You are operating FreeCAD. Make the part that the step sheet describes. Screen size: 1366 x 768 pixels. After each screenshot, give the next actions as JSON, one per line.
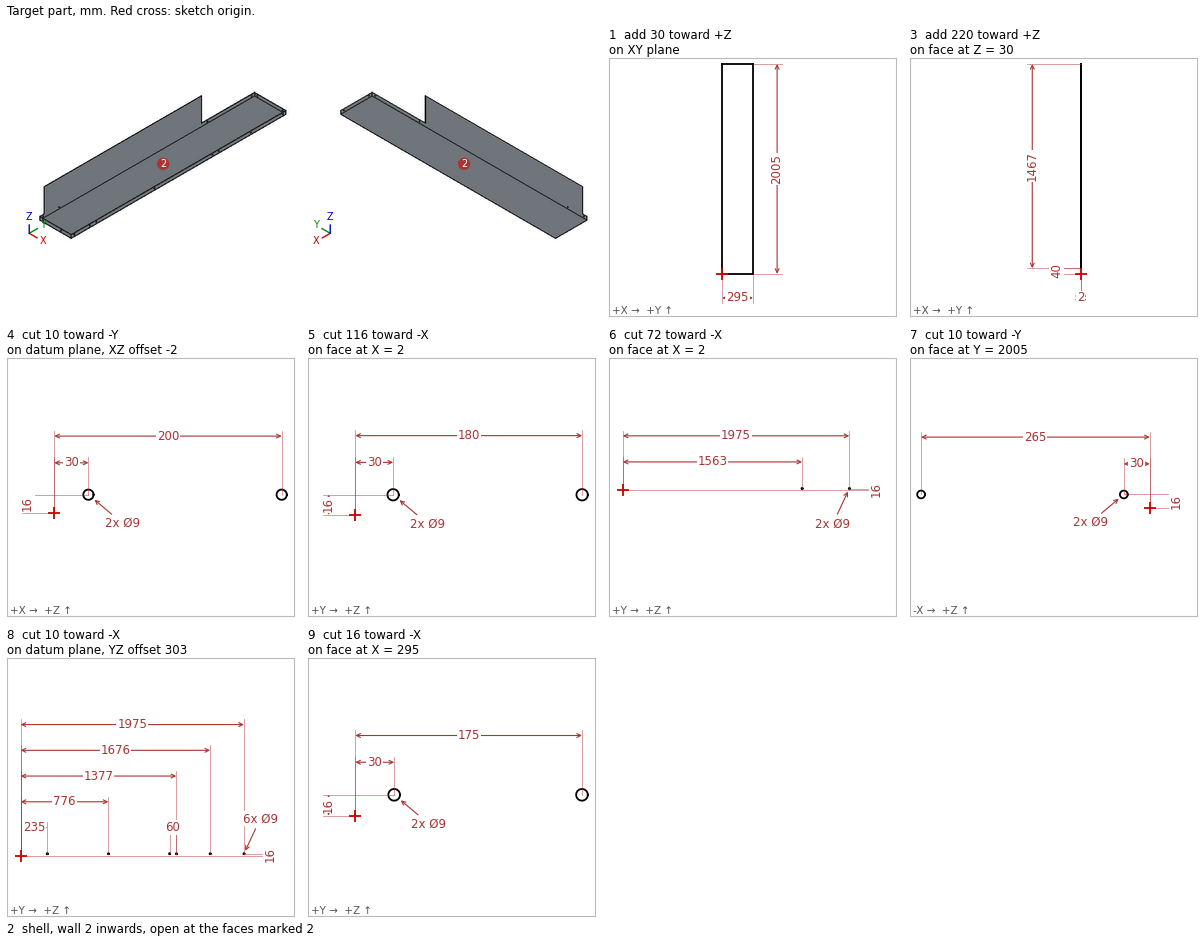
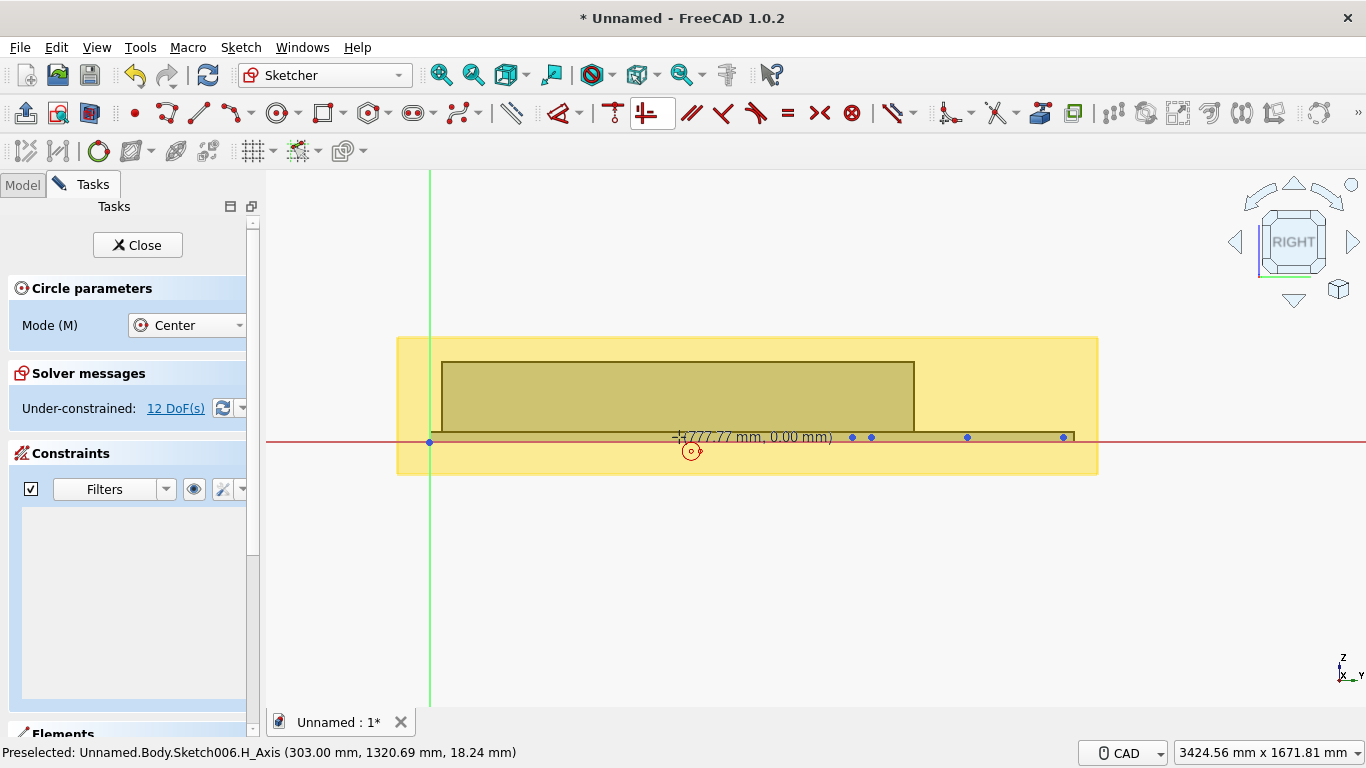
{"action": "scroll", "coordinate": [679, 437], "scroll_direction": "up", "scroll_amount": 6}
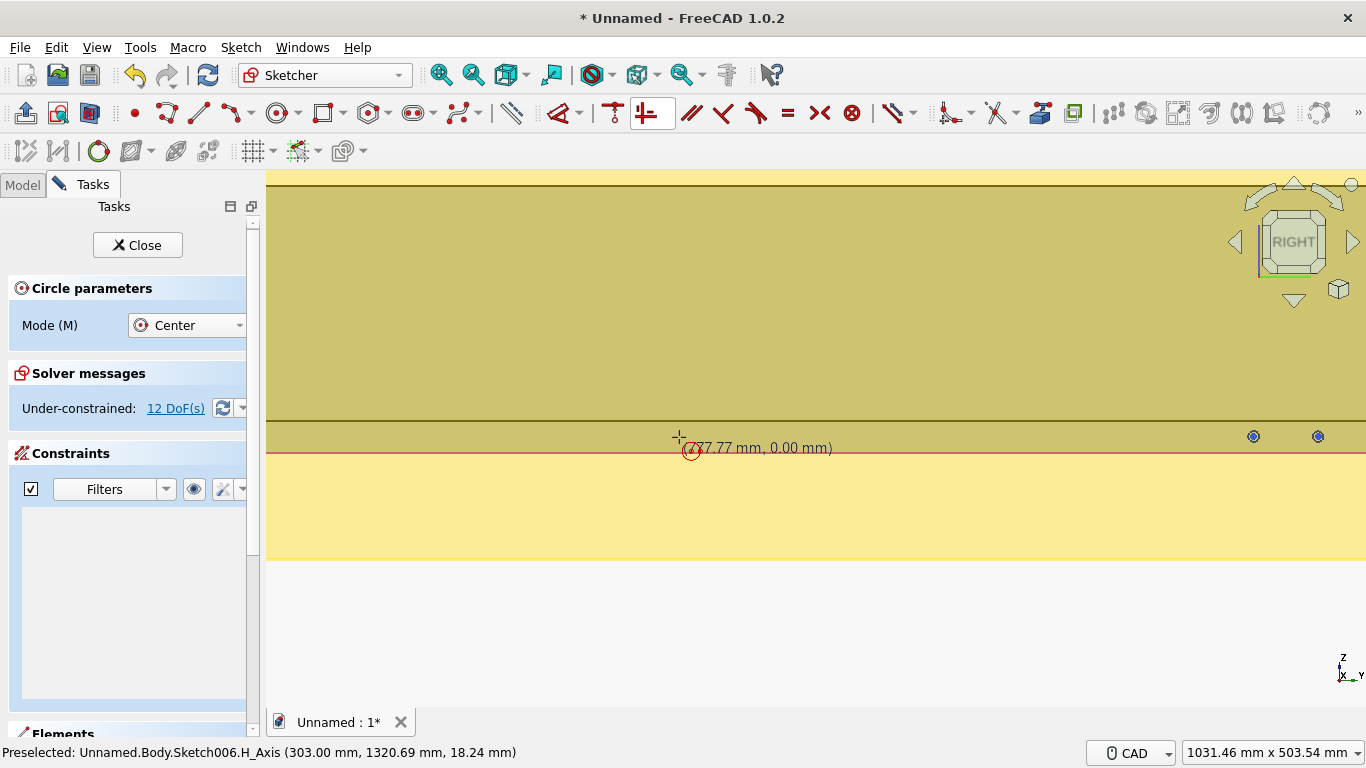
{"action": "left_click", "coordinate": [677, 436]}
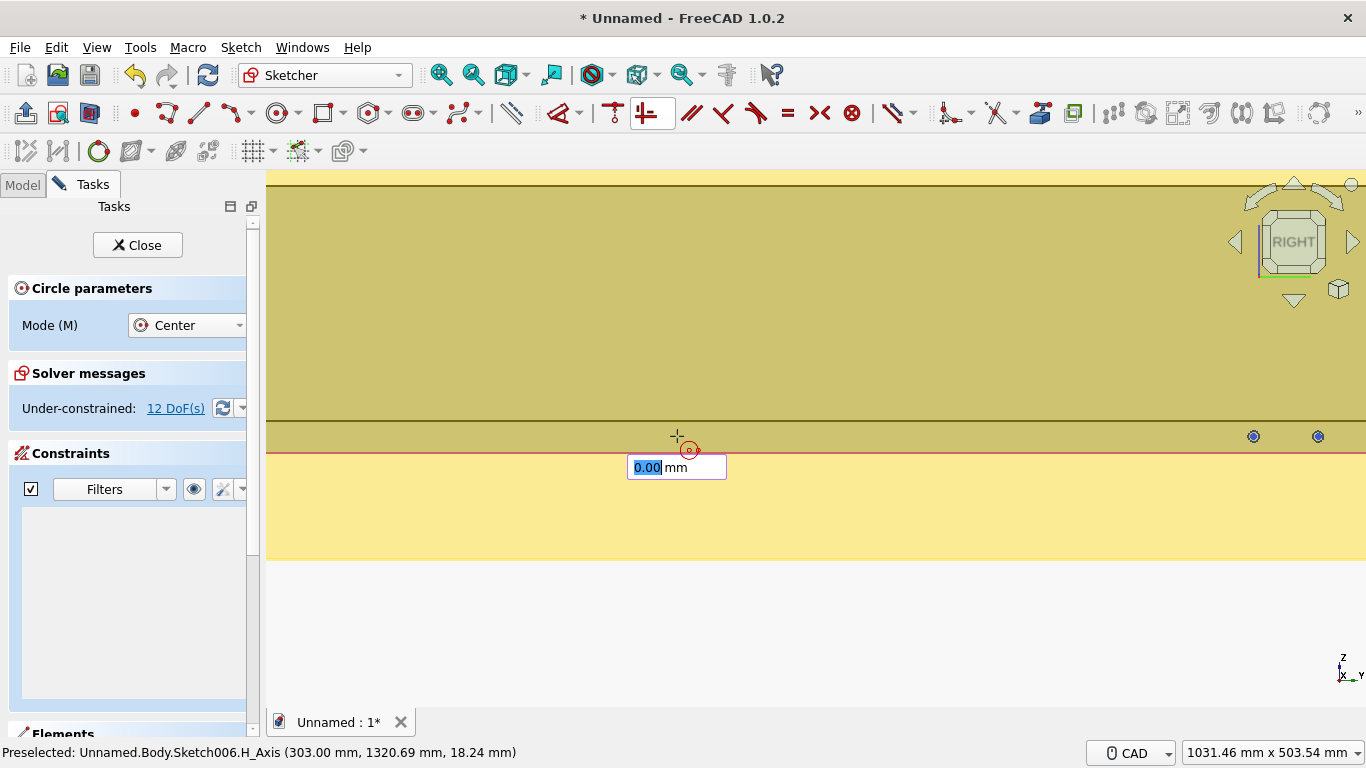
{"action": "scroll", "coordinate": [681, 432], "scroll_direction": "up", "scroll_amount": 6}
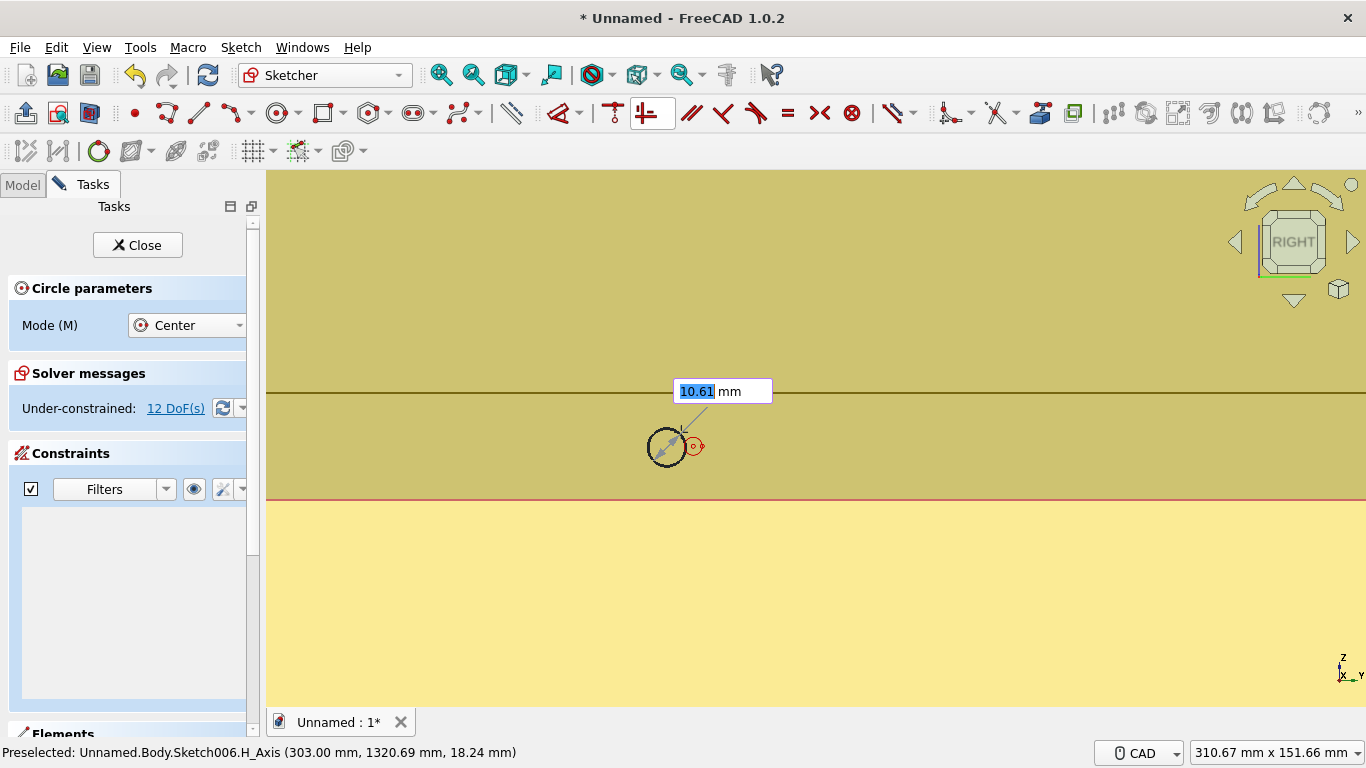
{"action": "left_click", "coordinate": [679, 432]}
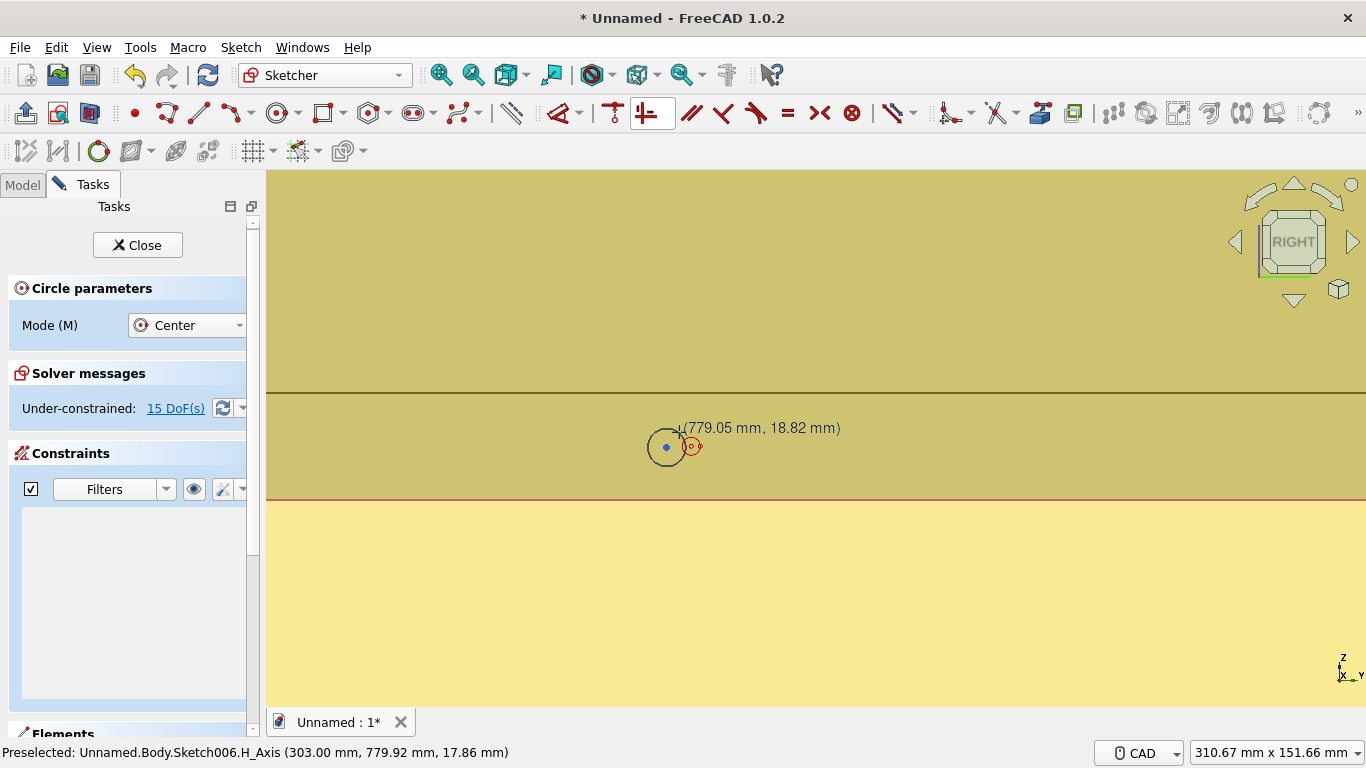
{"action": "scroll", "coordinate": [680, 436], "scroll_direction": "down", "scroll_amount": 12}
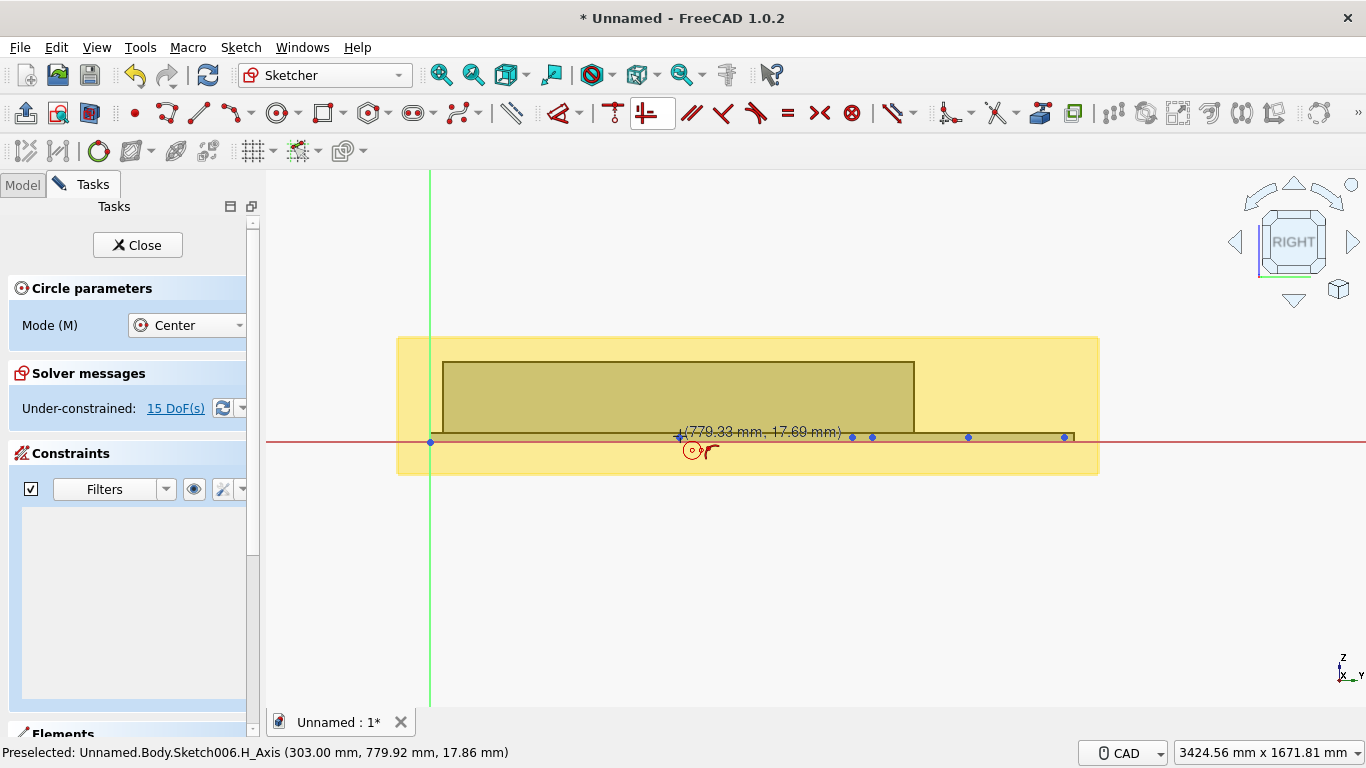
{"action": "scroll", "coordinate": [505, 437], "scroll_direction": "up", "scroll_amount": 14}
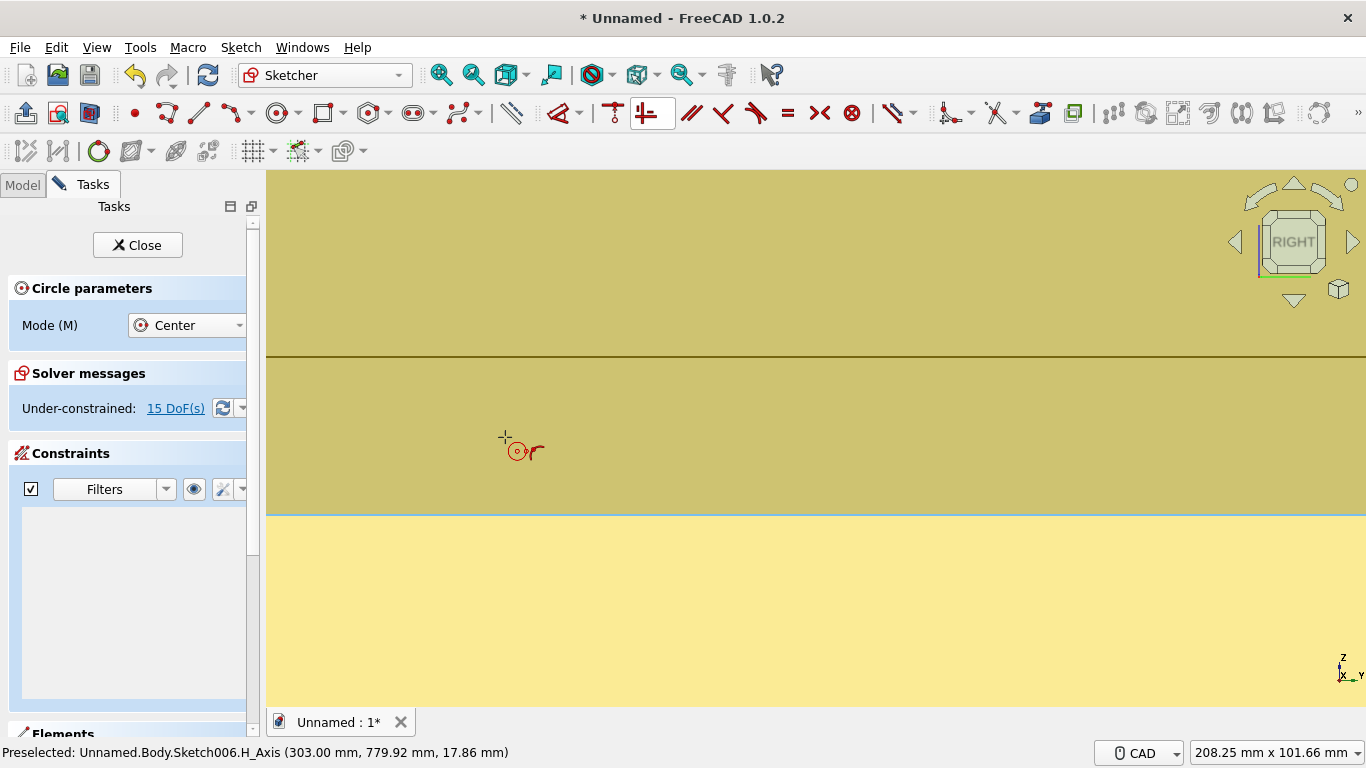
{"action": "scroll", "coordinate": [505, 437], "scroll_direction": "down", "scroll_amount": 14}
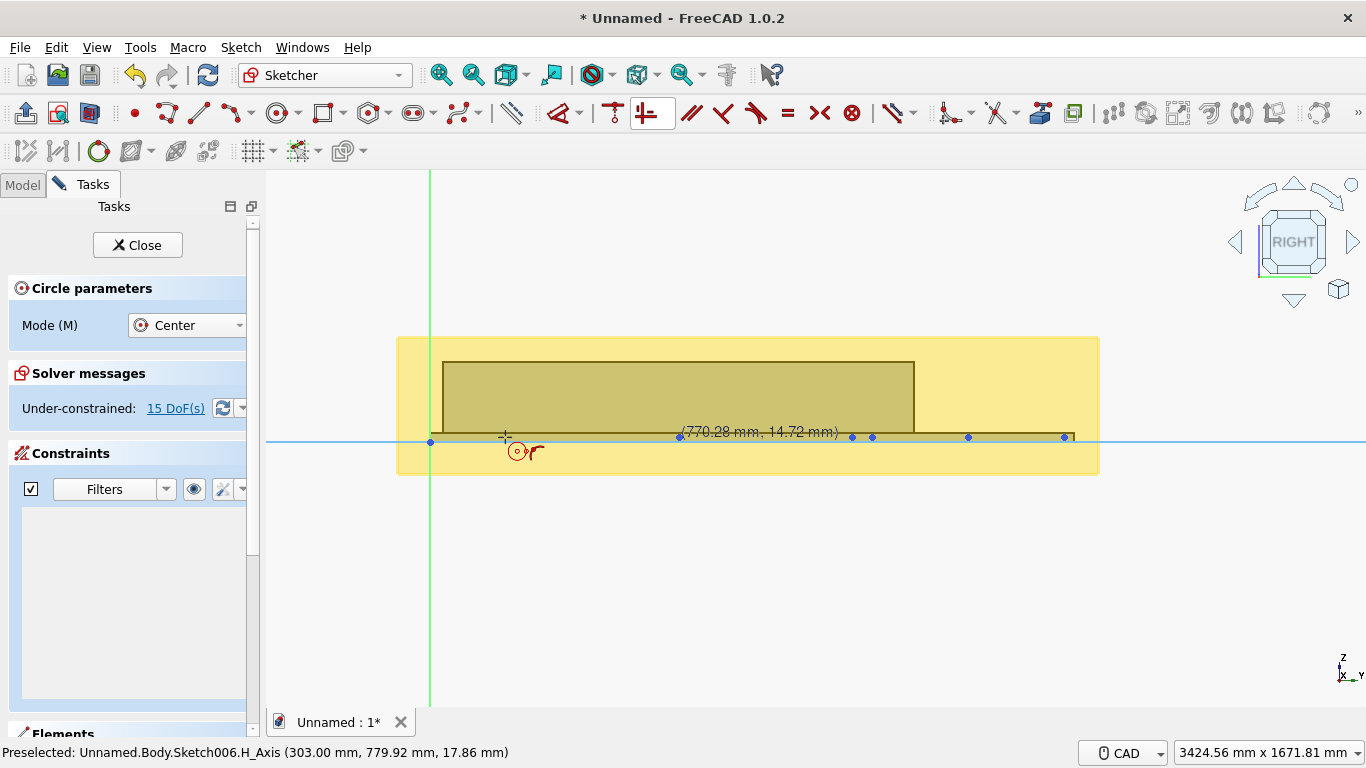
{"action": "scroll", "coordinate": [505, 437], "scroll_direction": "up", "scroll_amount": 6}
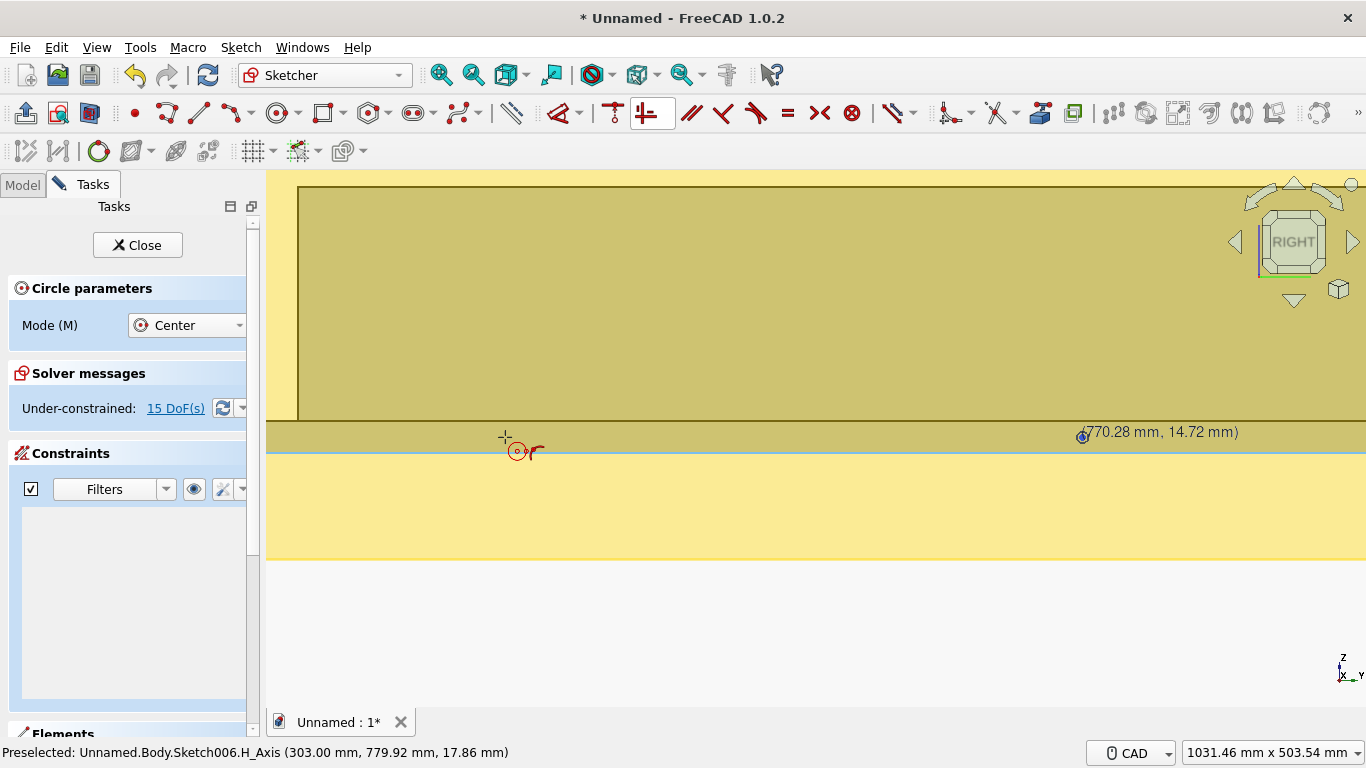
{"action": "left_click", "coordinate": [506, 436]}